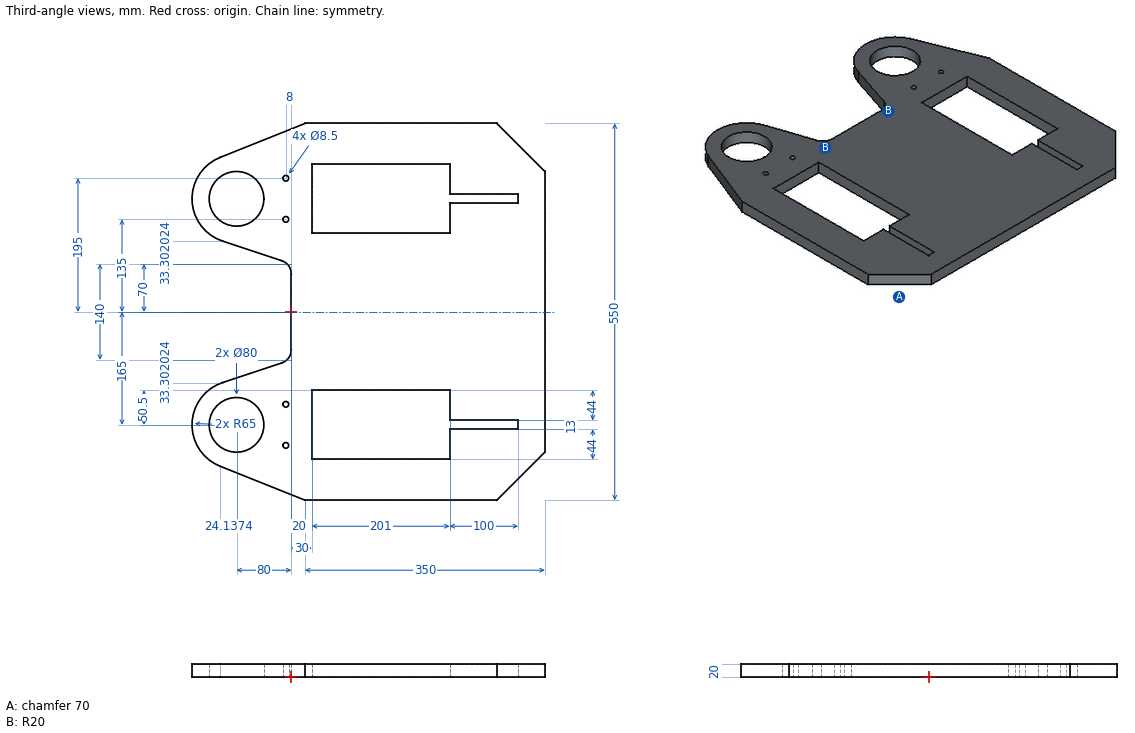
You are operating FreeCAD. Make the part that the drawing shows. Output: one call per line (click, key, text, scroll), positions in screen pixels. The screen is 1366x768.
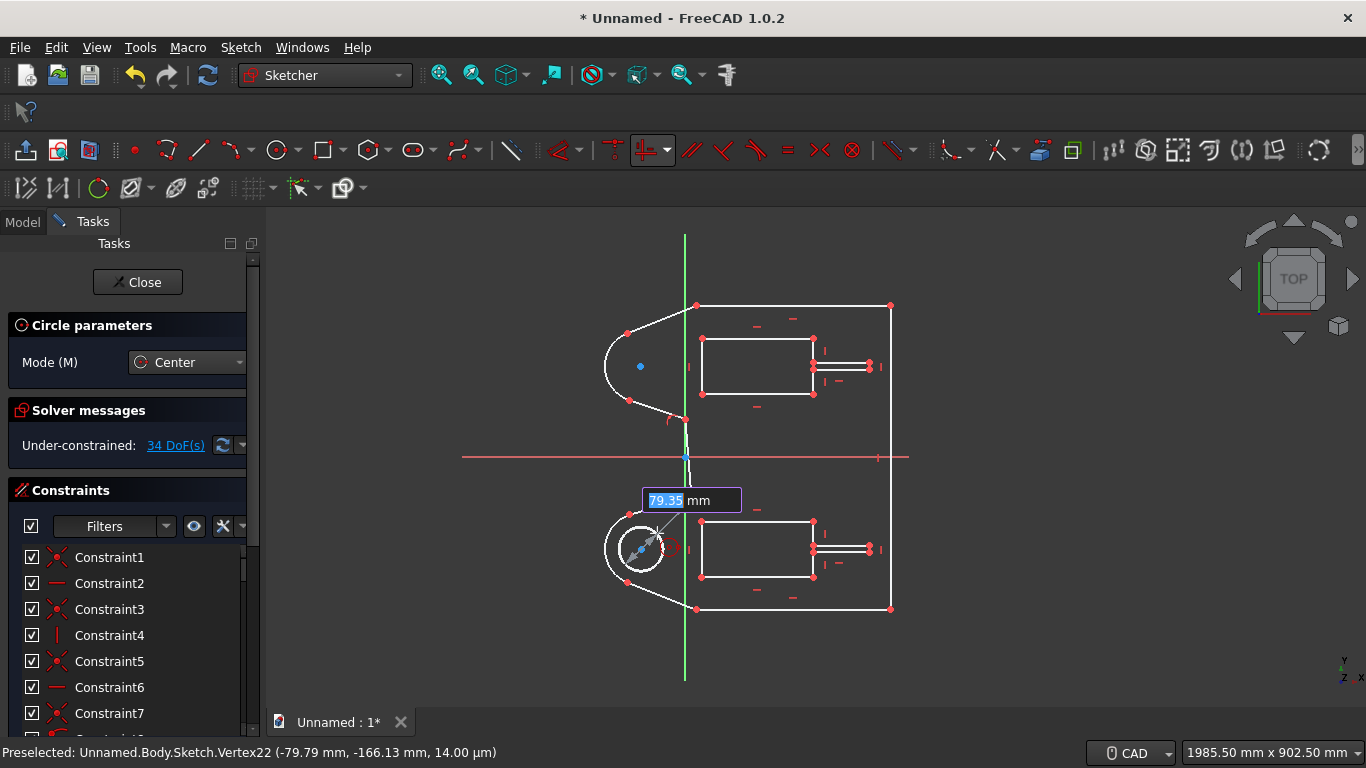
text(80)
key(Return)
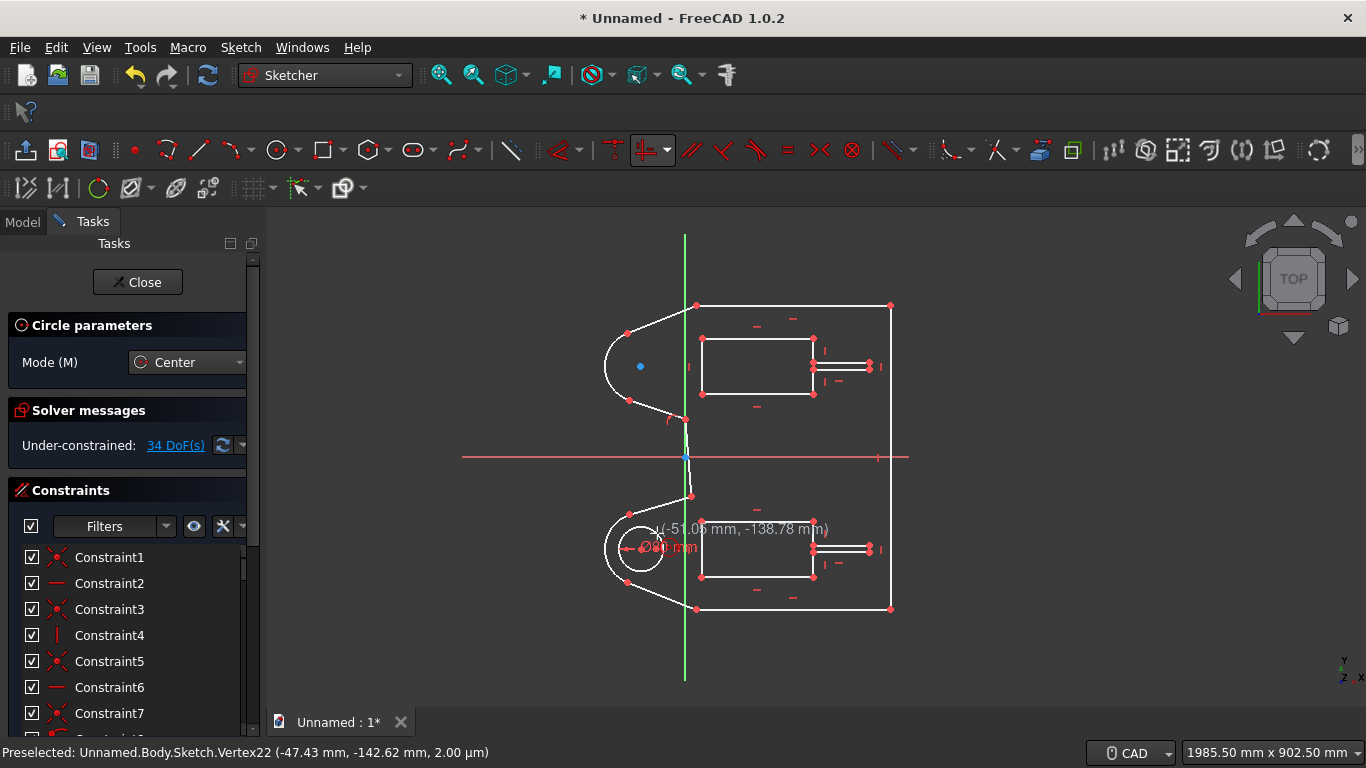
click(641, 366)
move(657, 350)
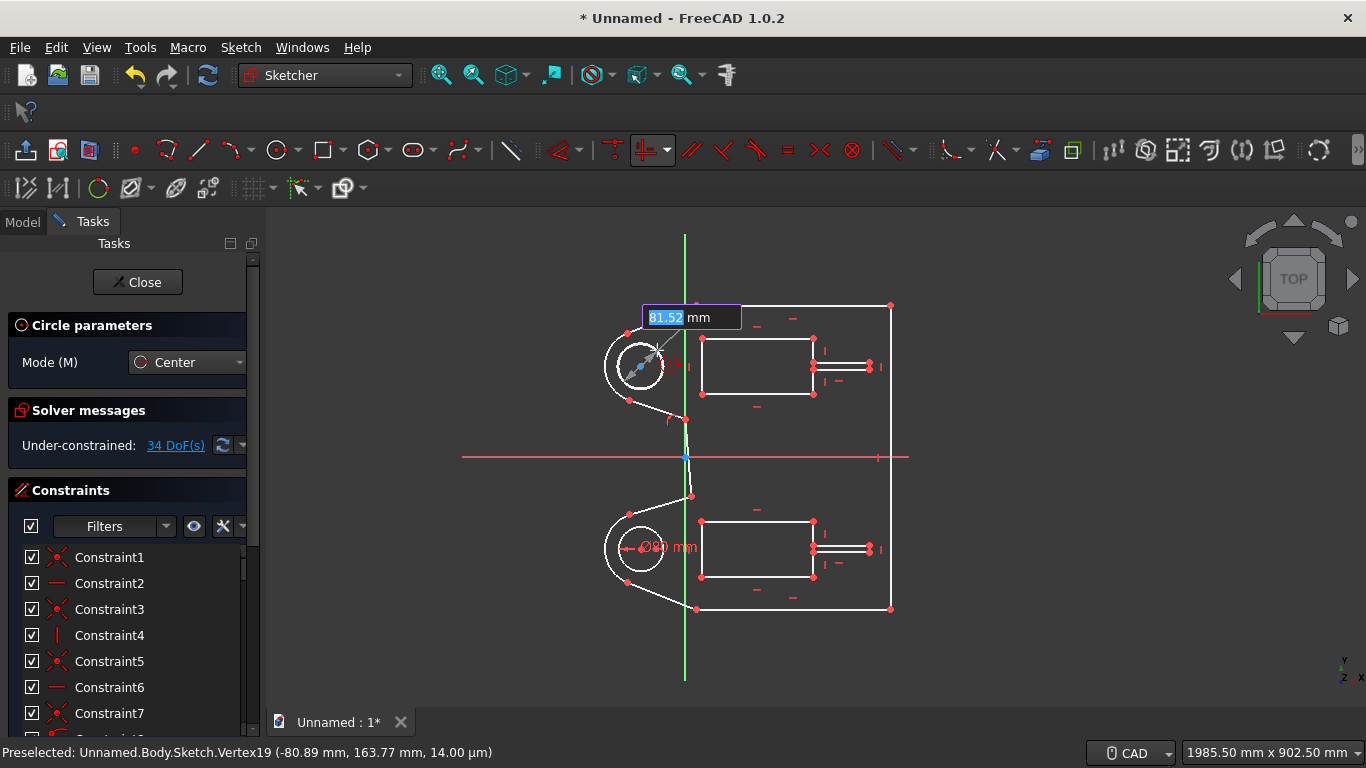
text(80)
key(Return)
key(Escape)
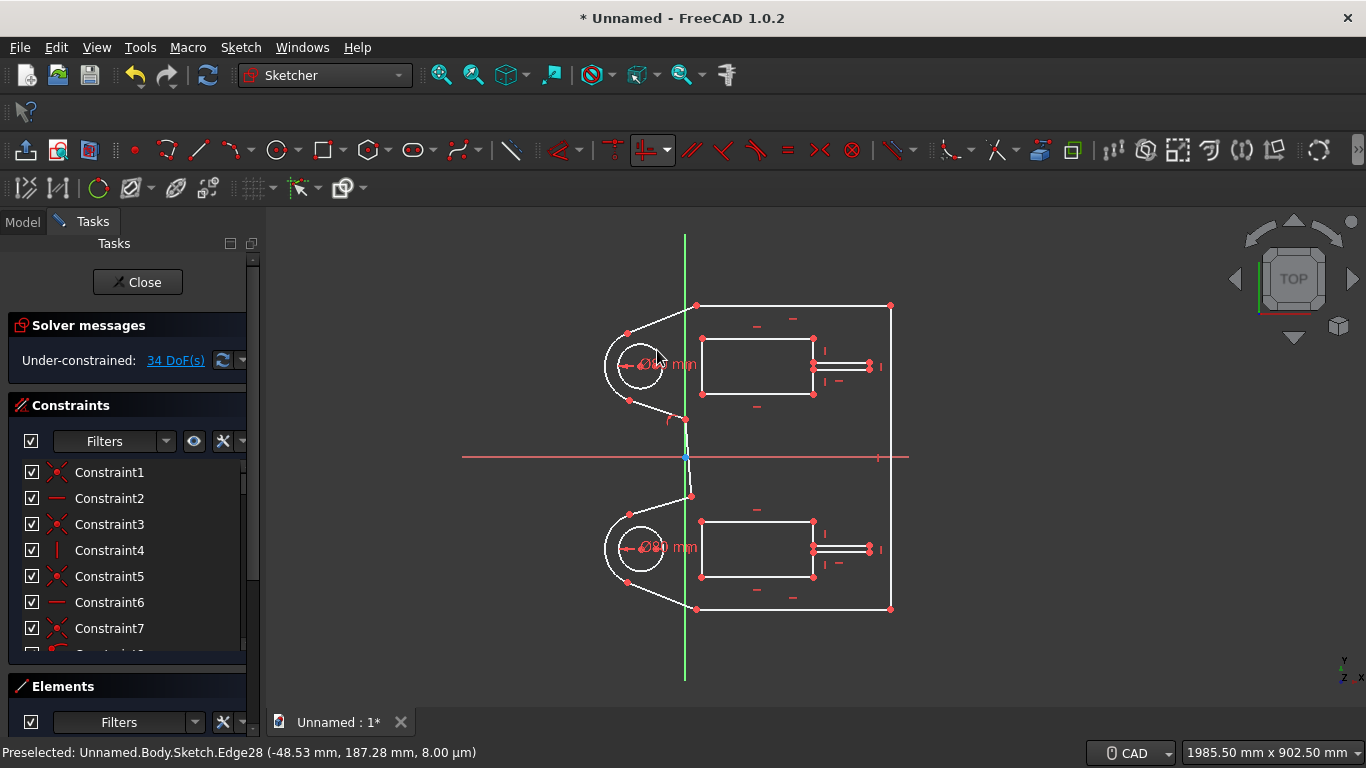
click(687, 442)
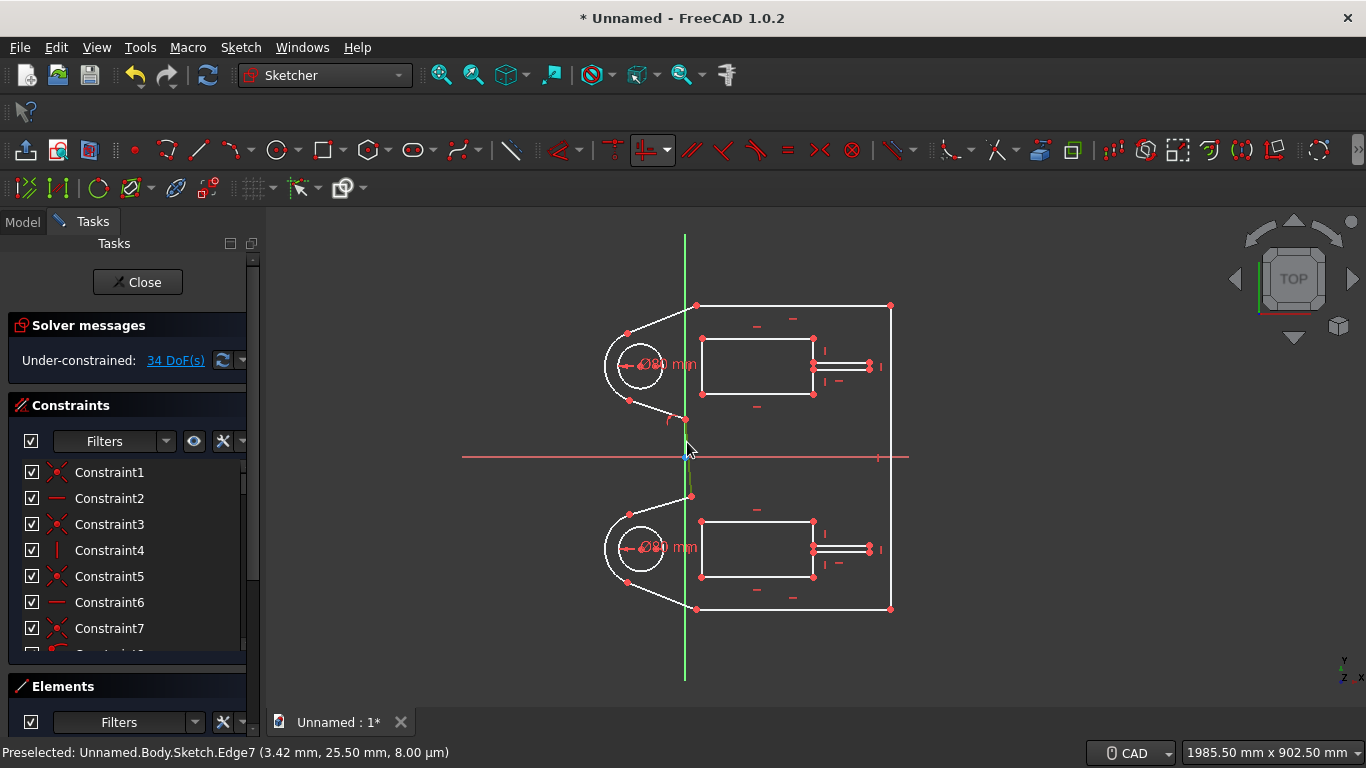
key(v)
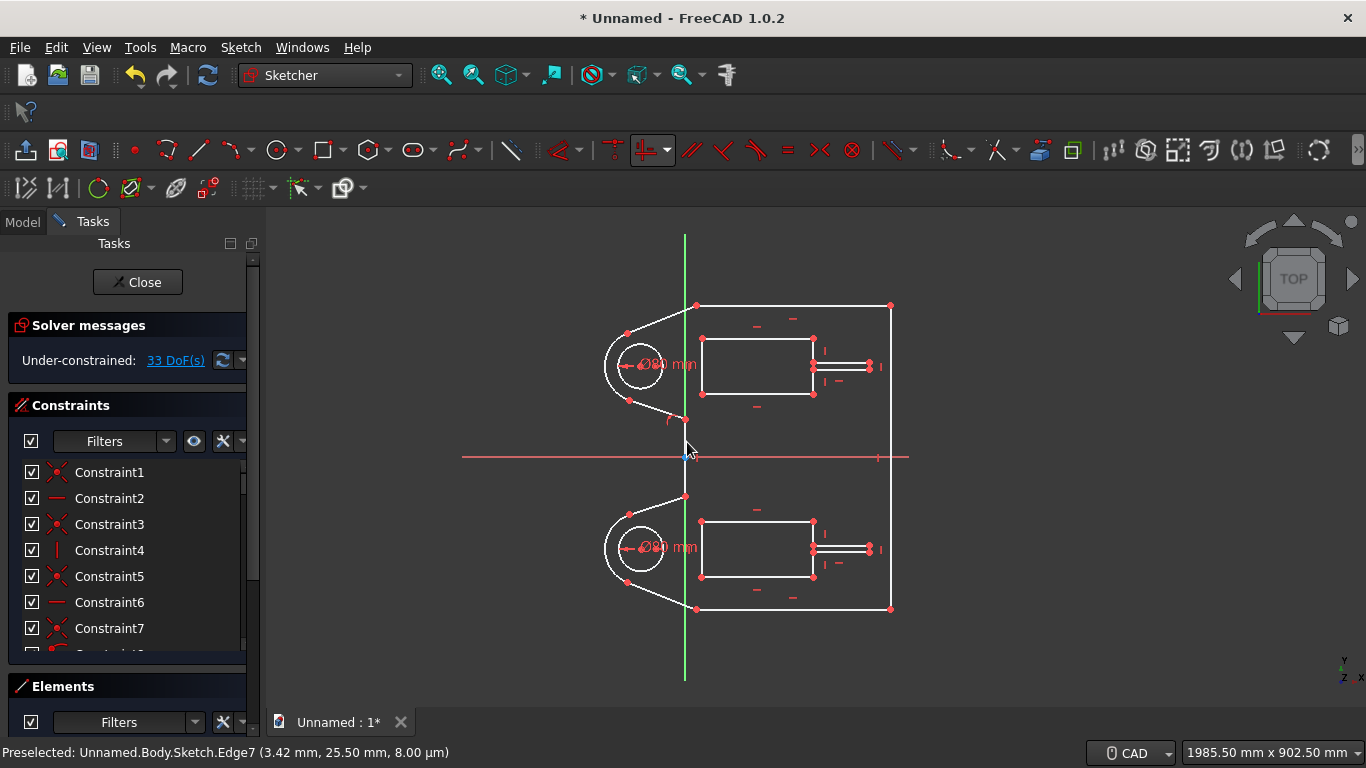
click(609, 350)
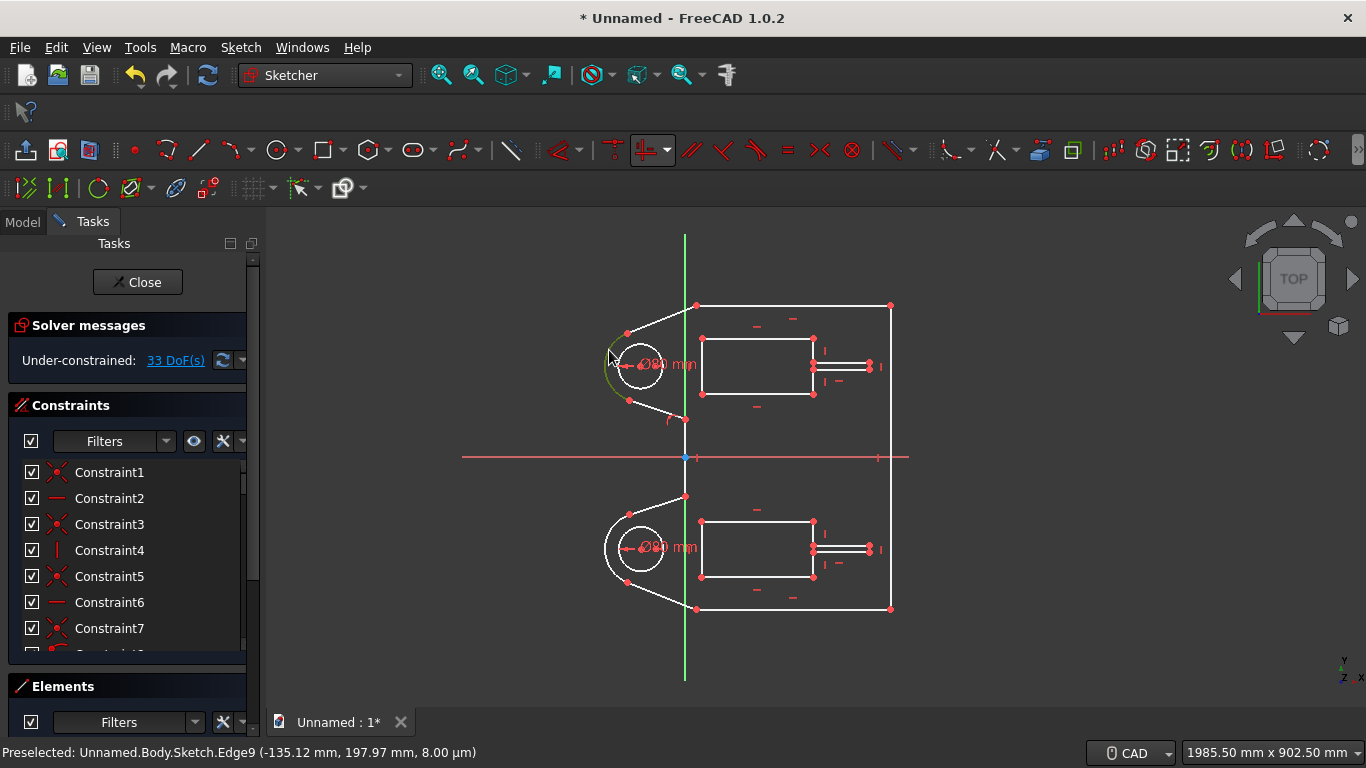
click(610, 531)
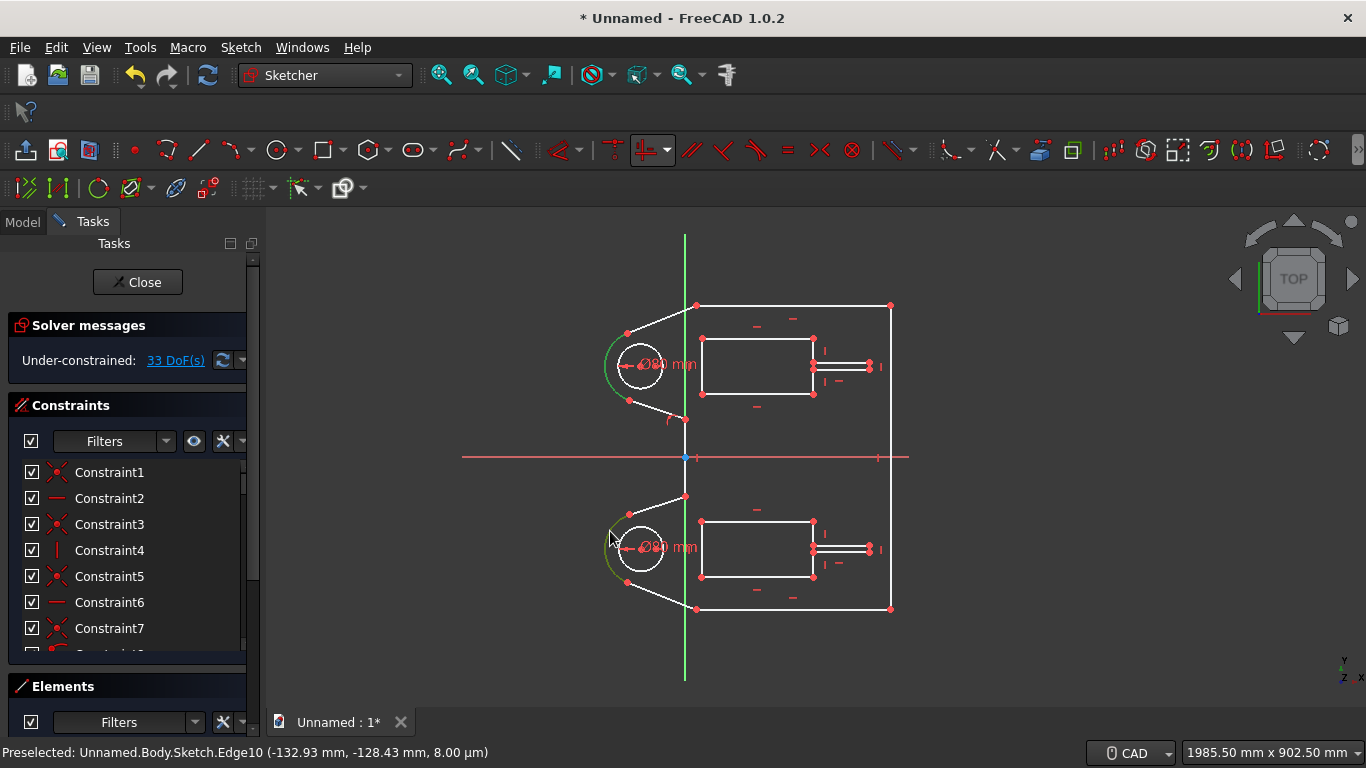
key(e)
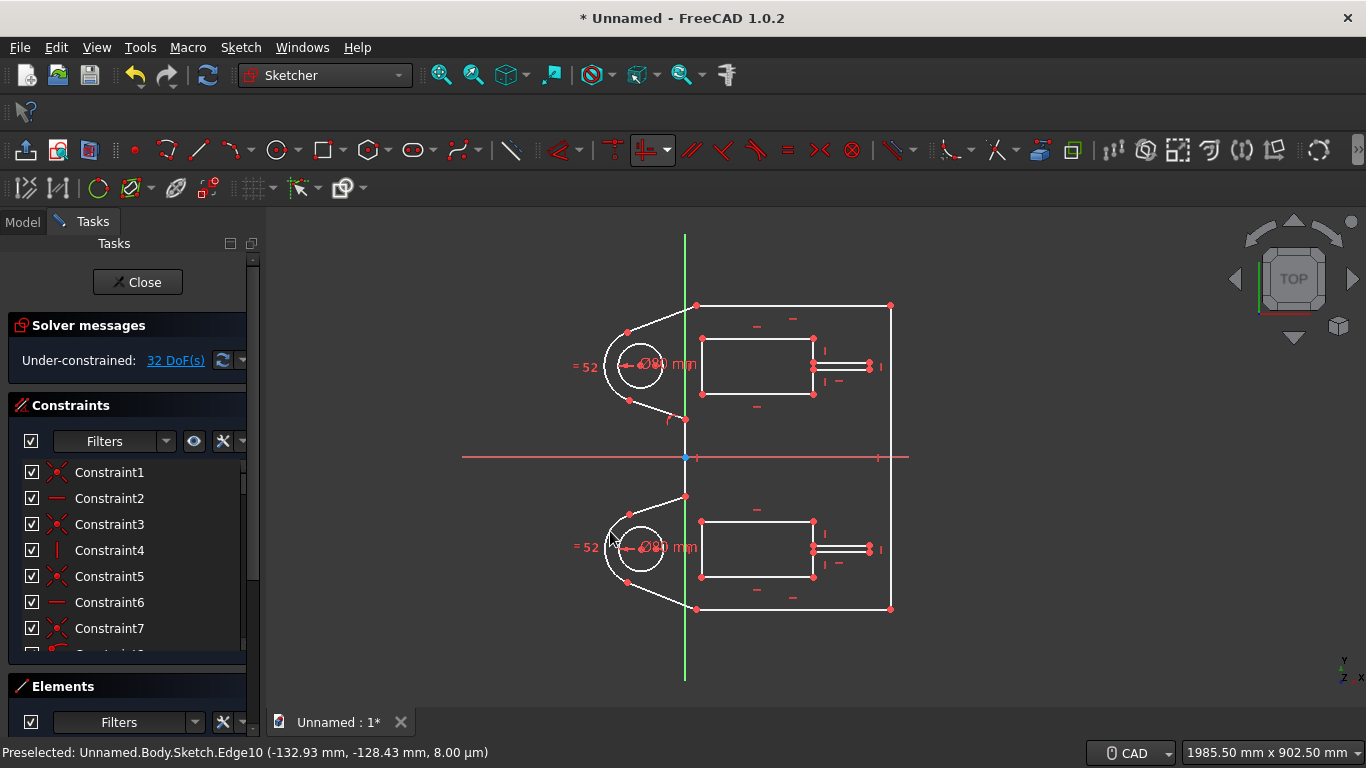
click(640, 366)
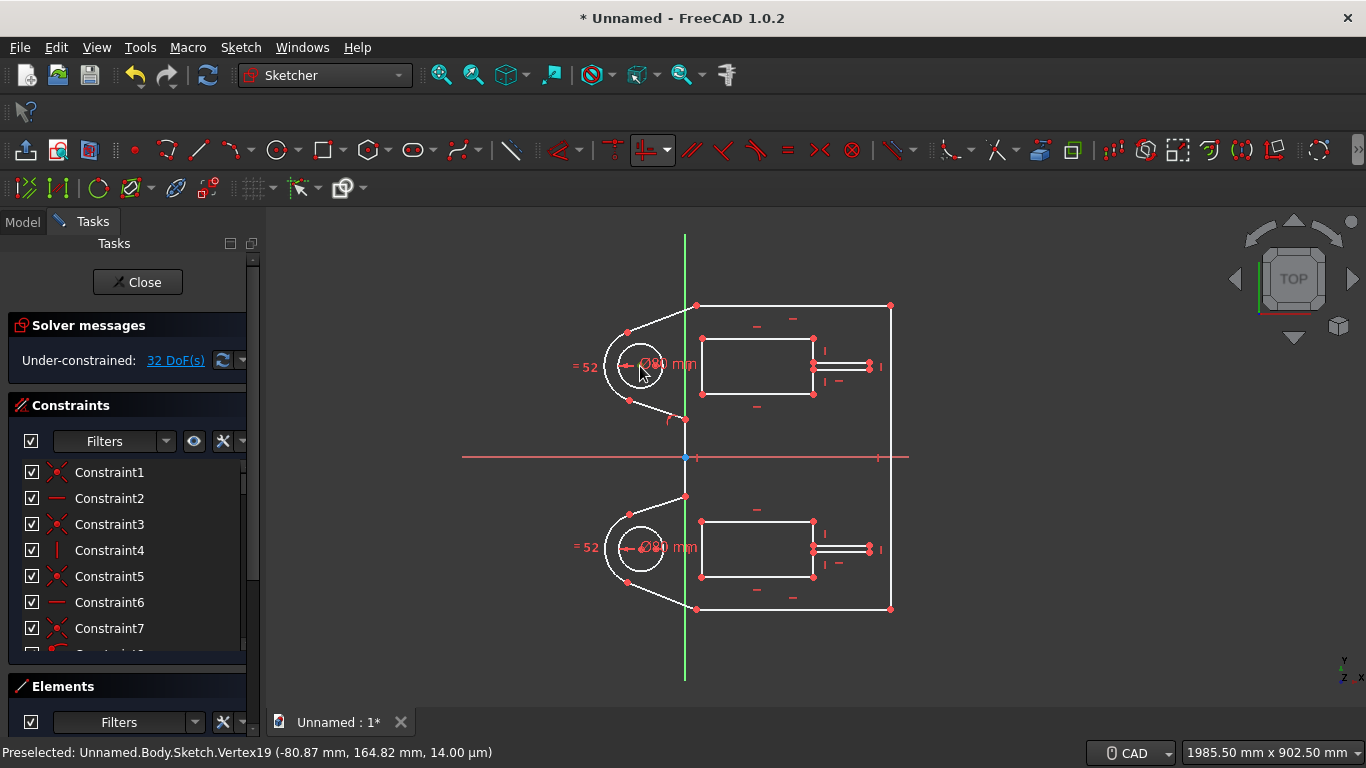
click(641, 549)